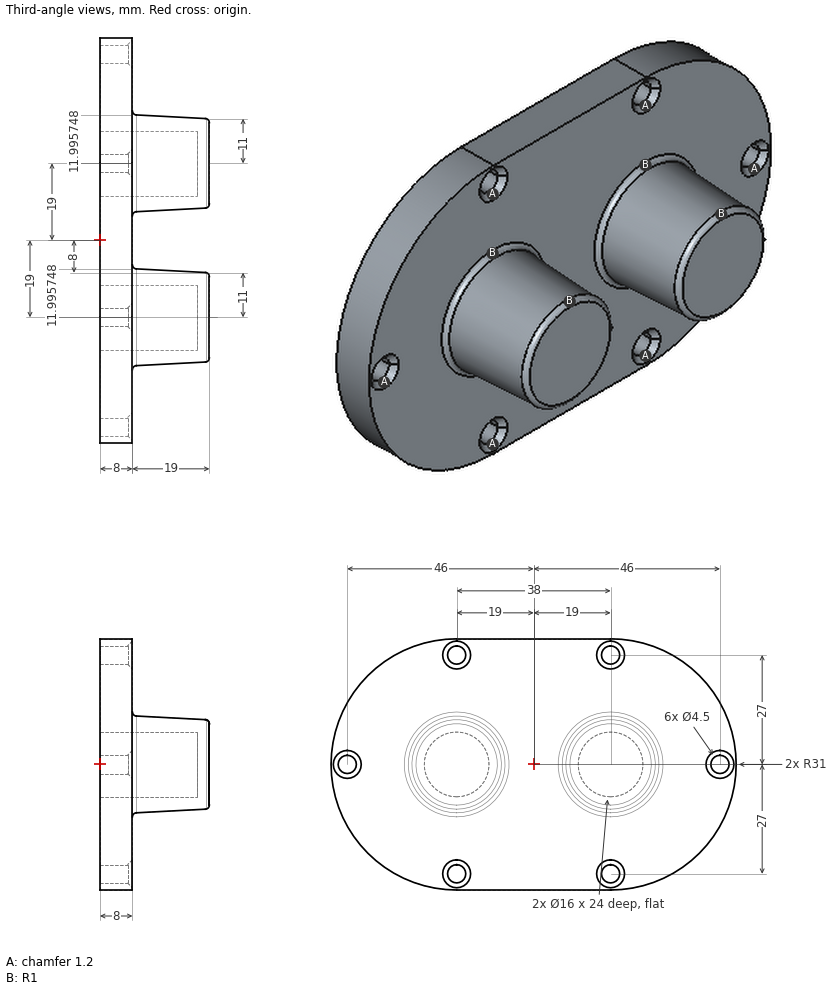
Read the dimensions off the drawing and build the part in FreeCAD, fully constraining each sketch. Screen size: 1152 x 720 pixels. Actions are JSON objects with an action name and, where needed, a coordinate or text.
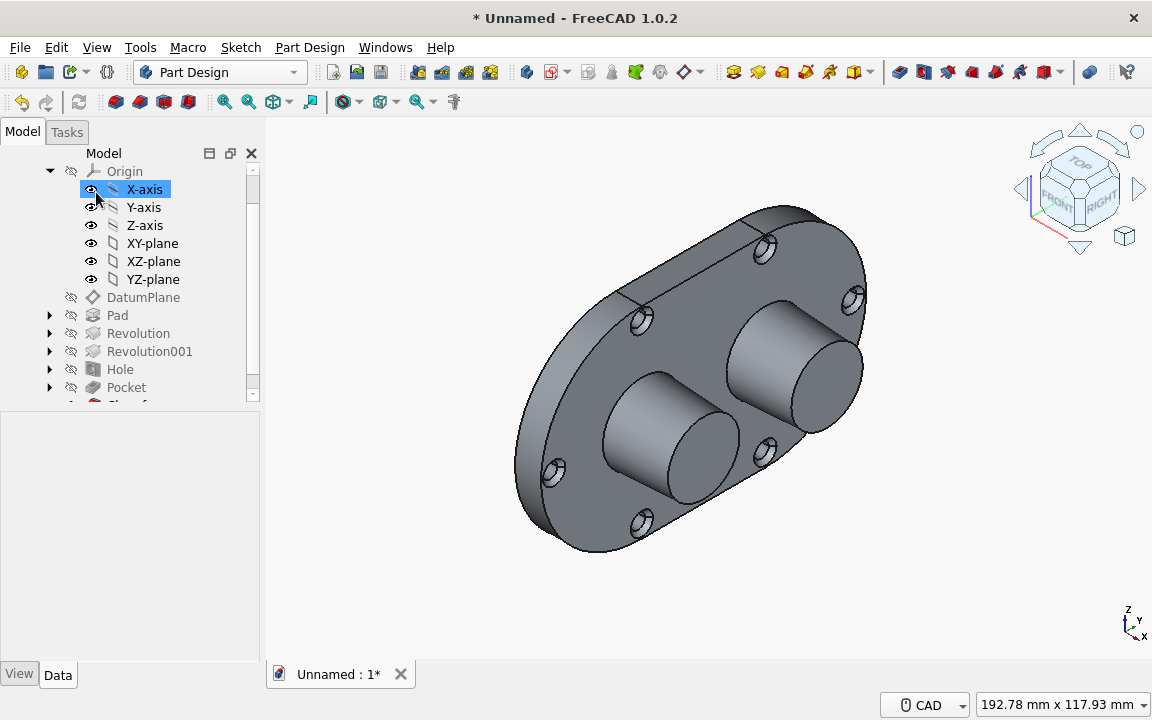
{"action": "left_click", "coordinate": [668, 478]}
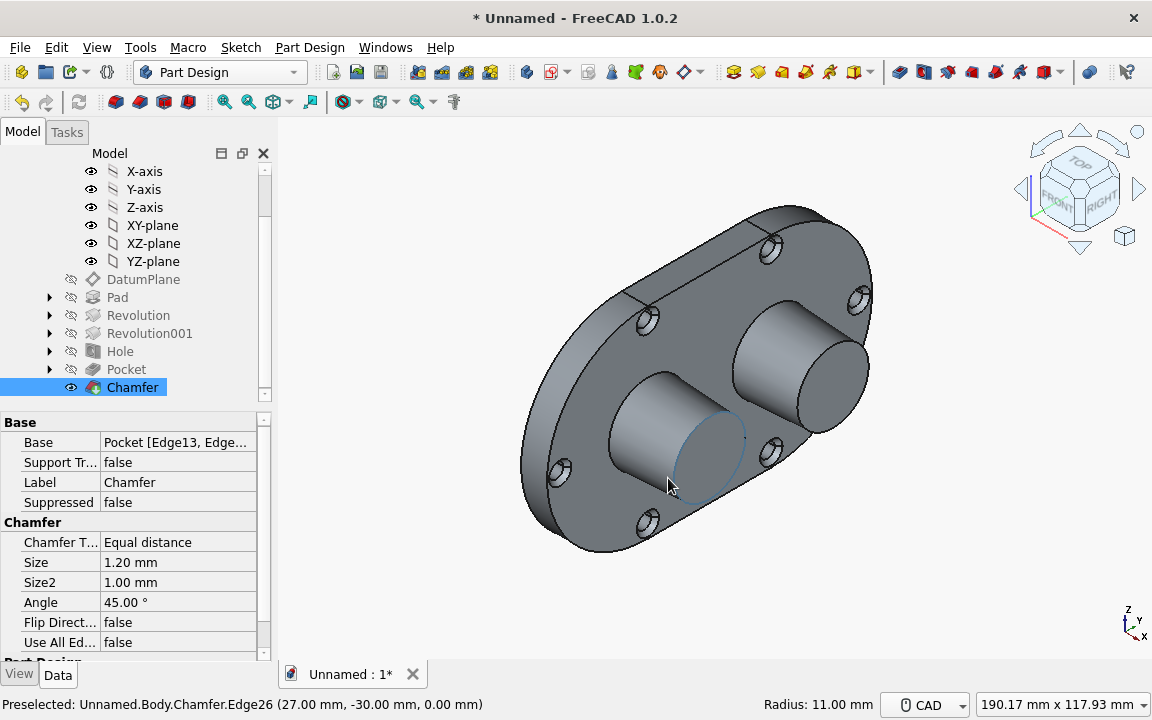
{"action": "left_click", "coordinate": [797, 406], "text": "ctrl"}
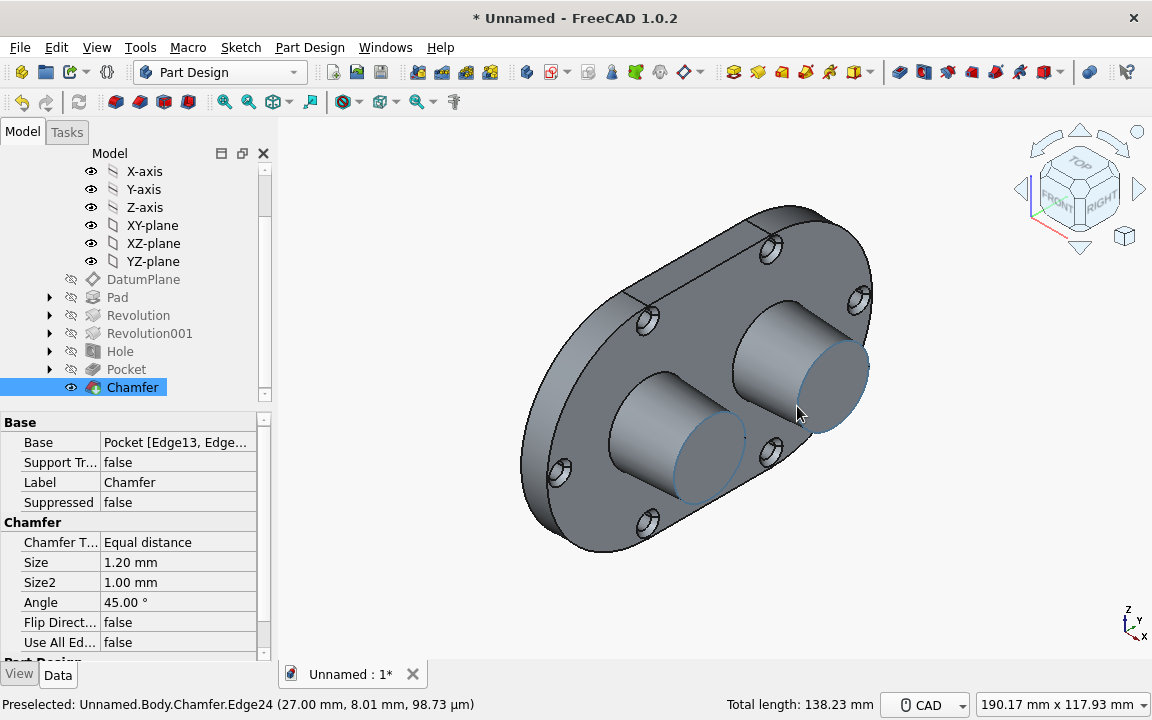
{"action": "key", "text": "2"}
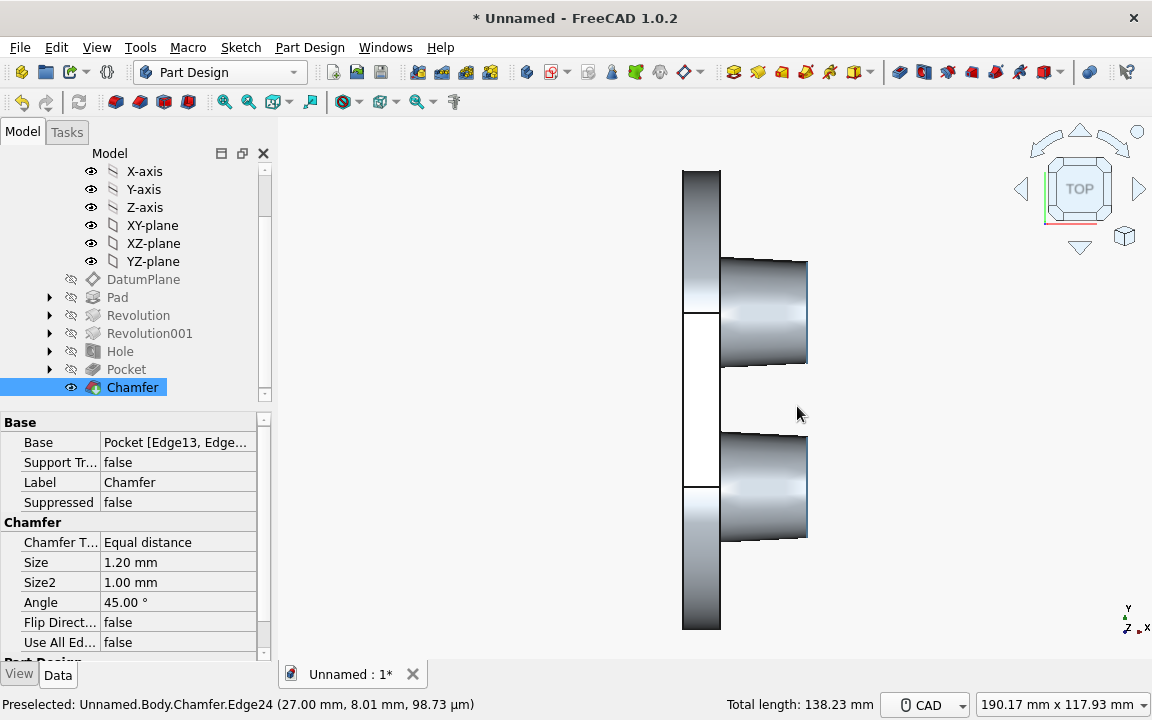
{"action": "key", "text": "0"}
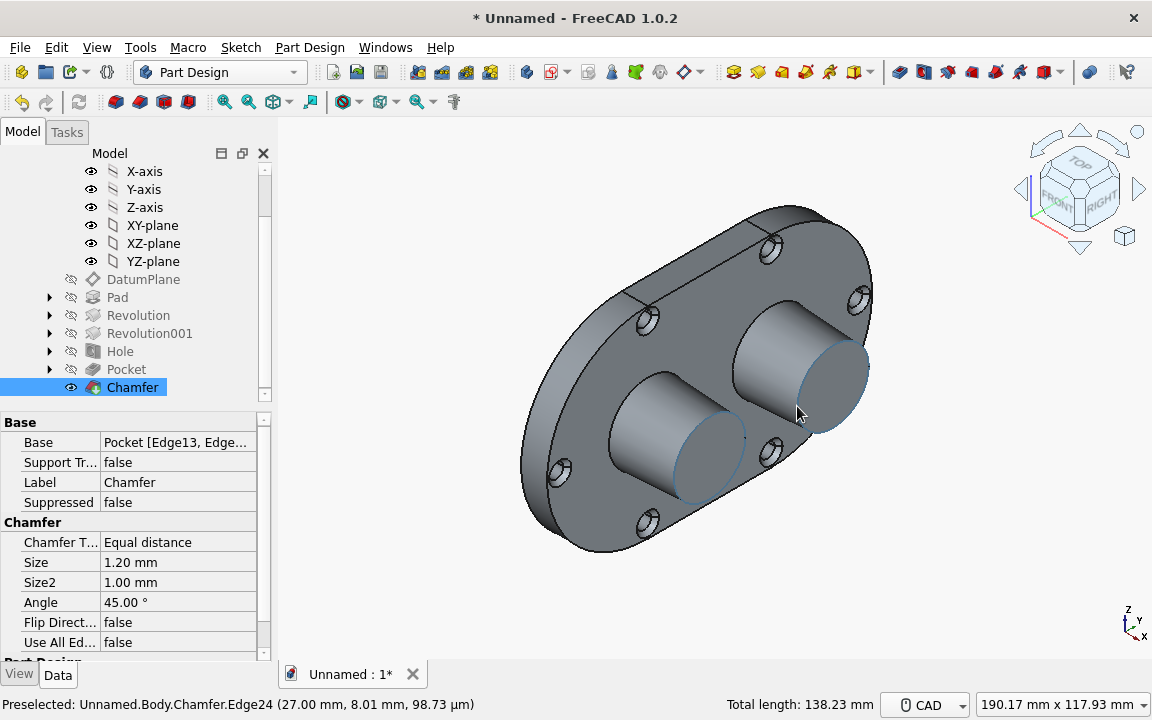
{"action": "key", "text": "1"}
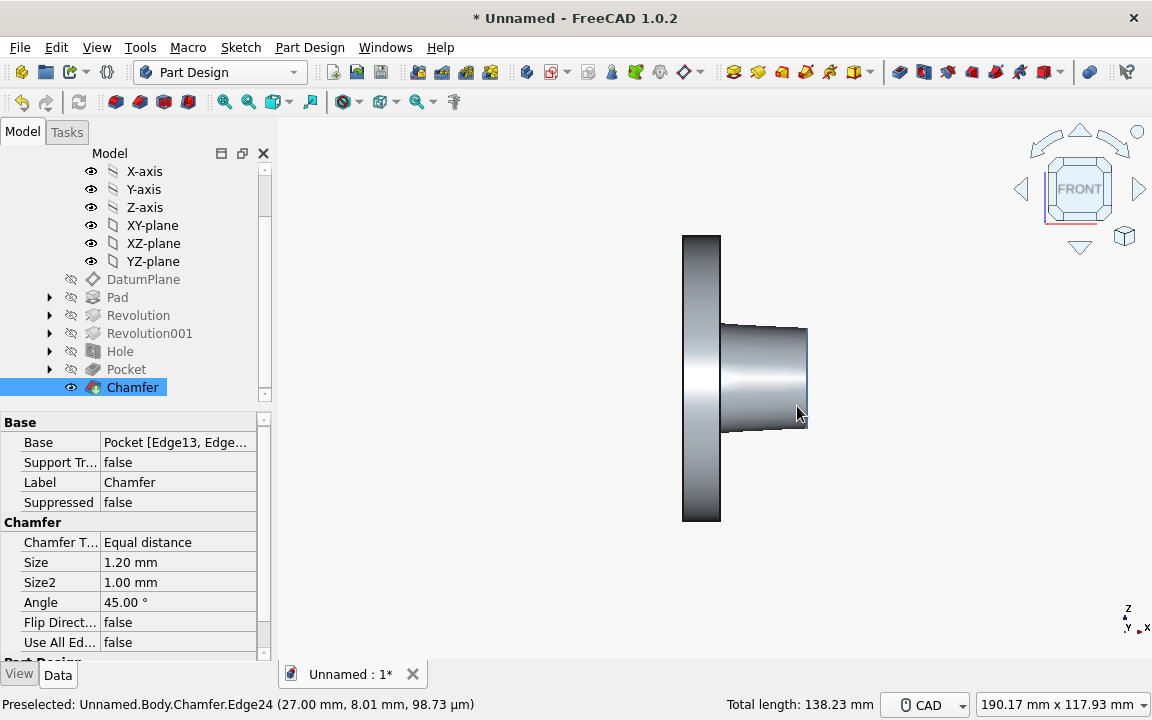
{"action": "key", "text": "3"}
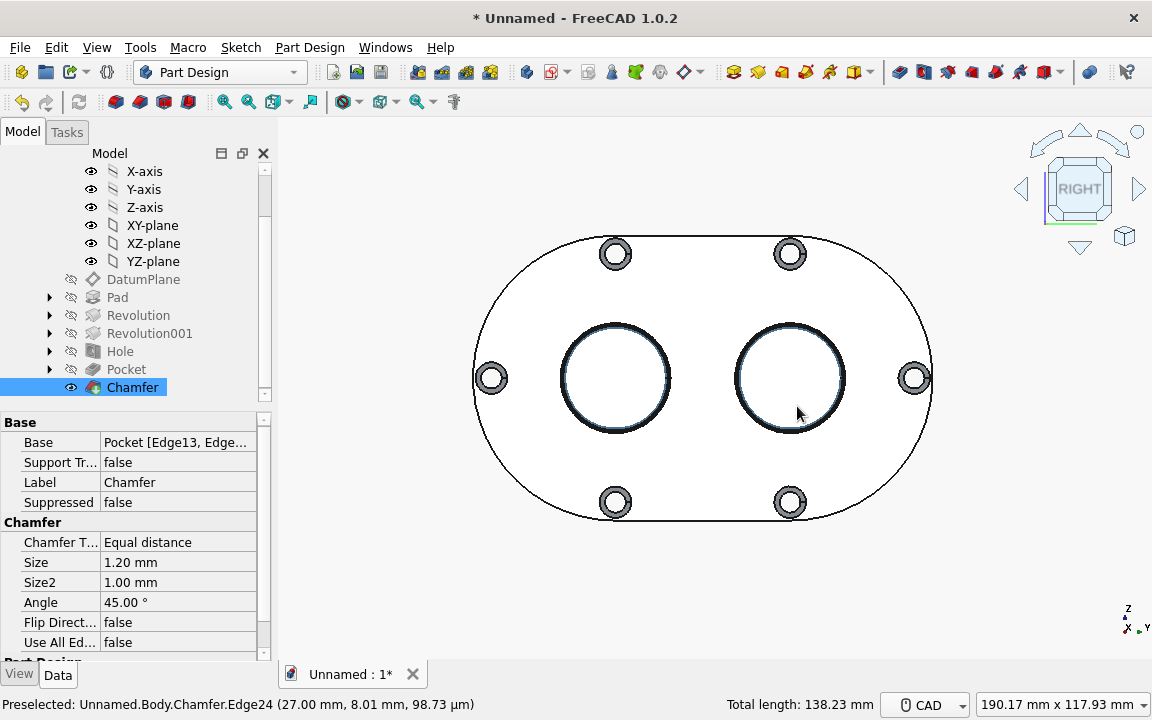
{"action": "key", "text": "5"}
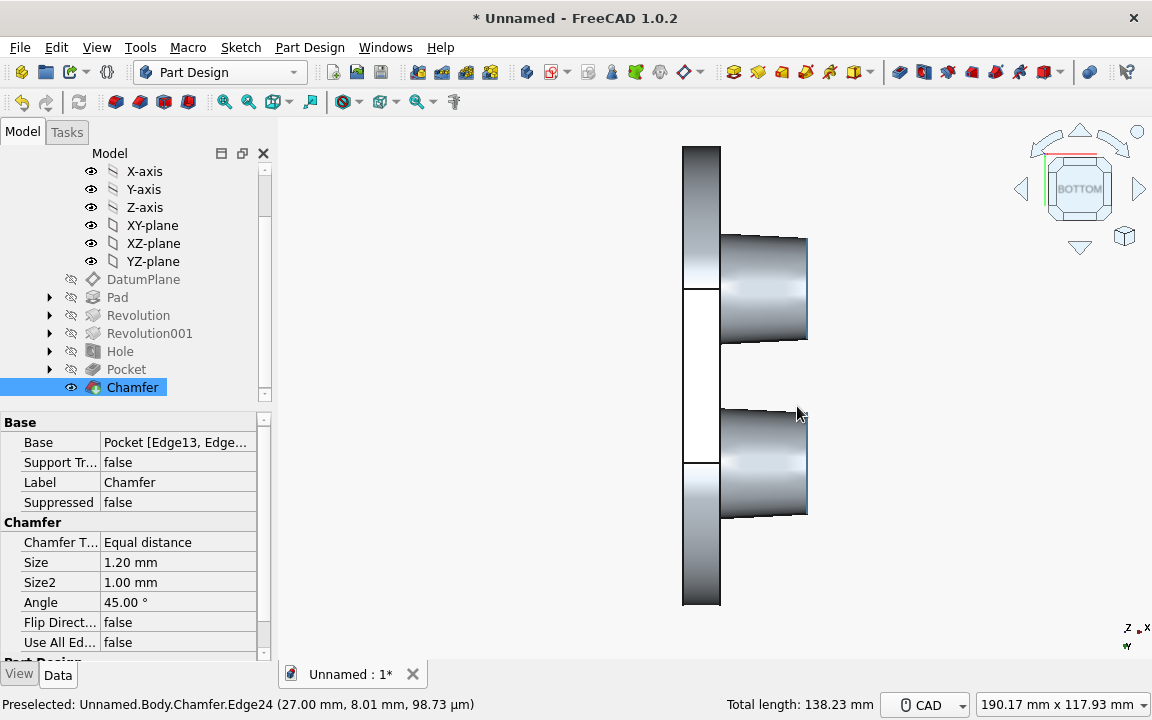
{"action": "key", "text": "4"}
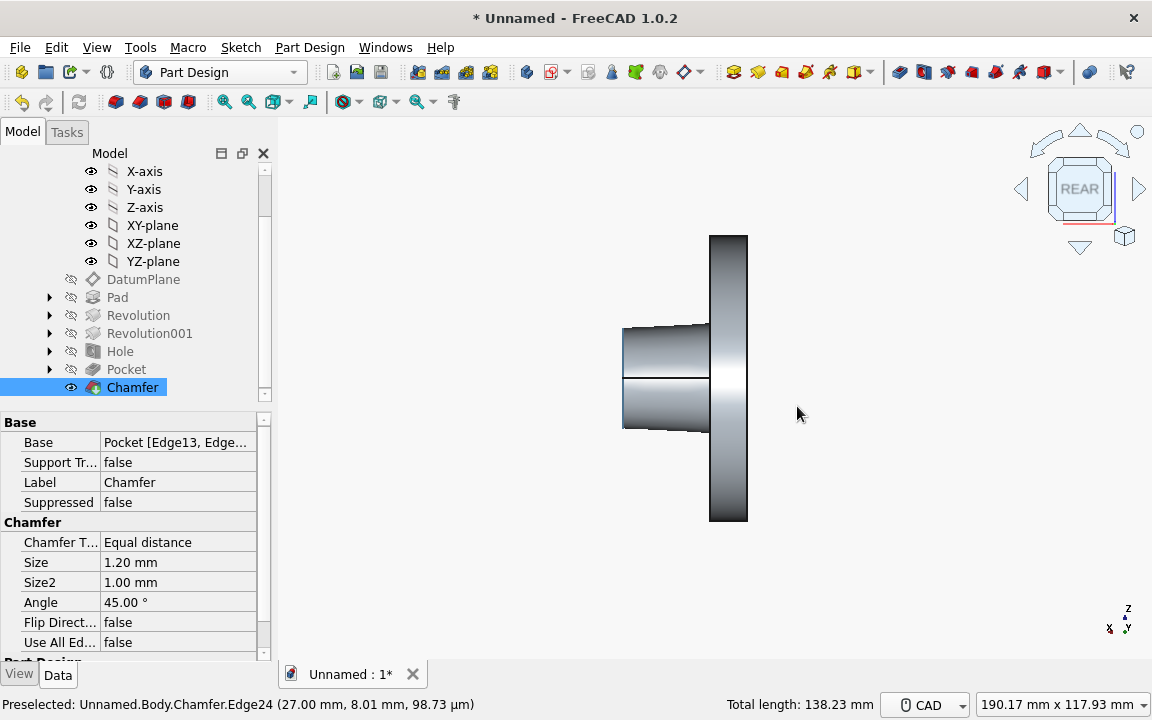
{"action": "key", "text": "6"}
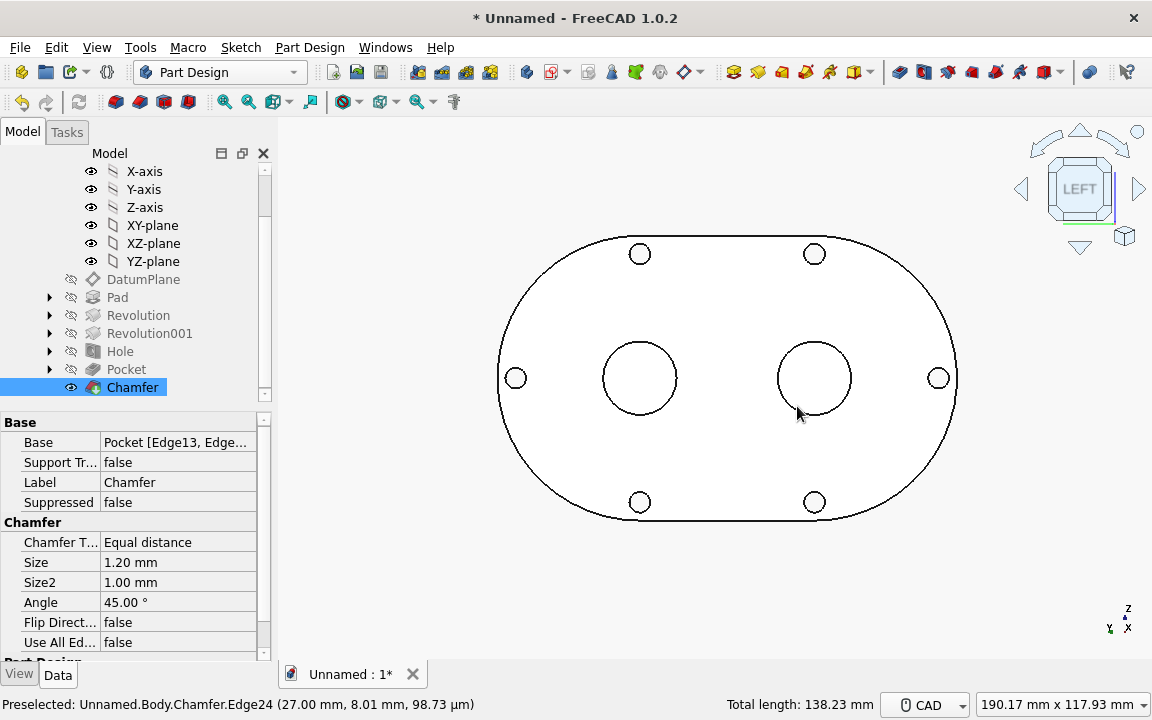
{"action": "key", "text": "v 3"}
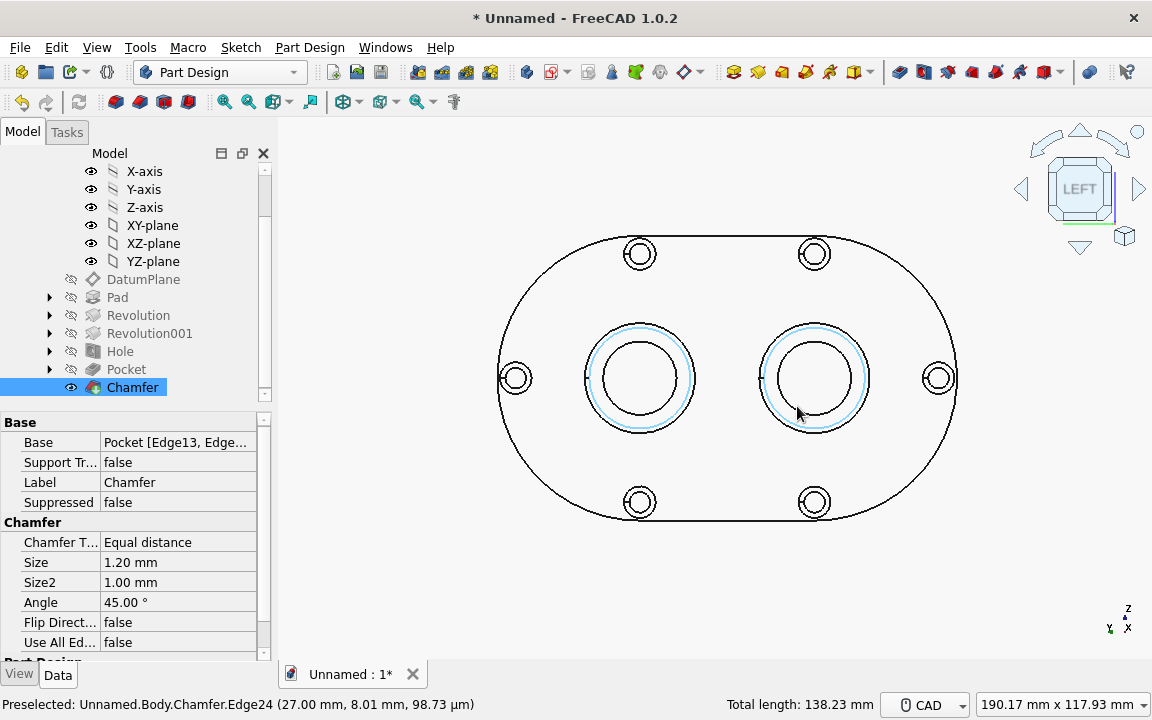
{"action": "key", "text": "0"}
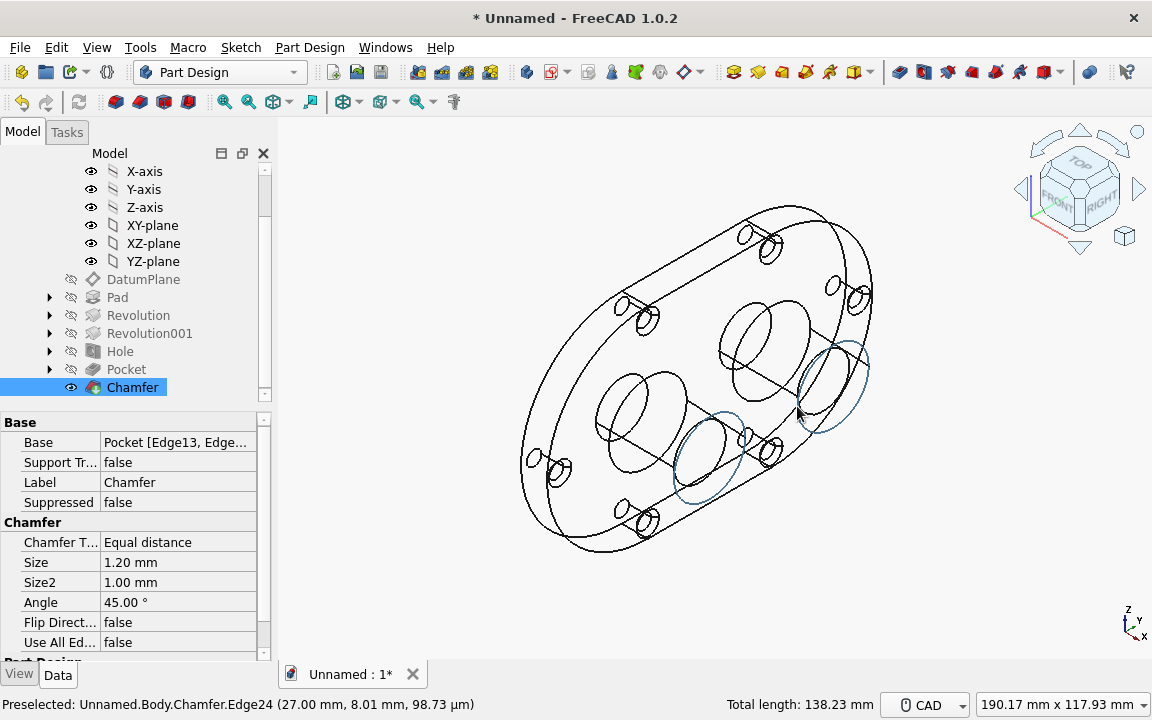
{"action": "left_click", "coordinate": [609, 444], "text": "ctrl"}